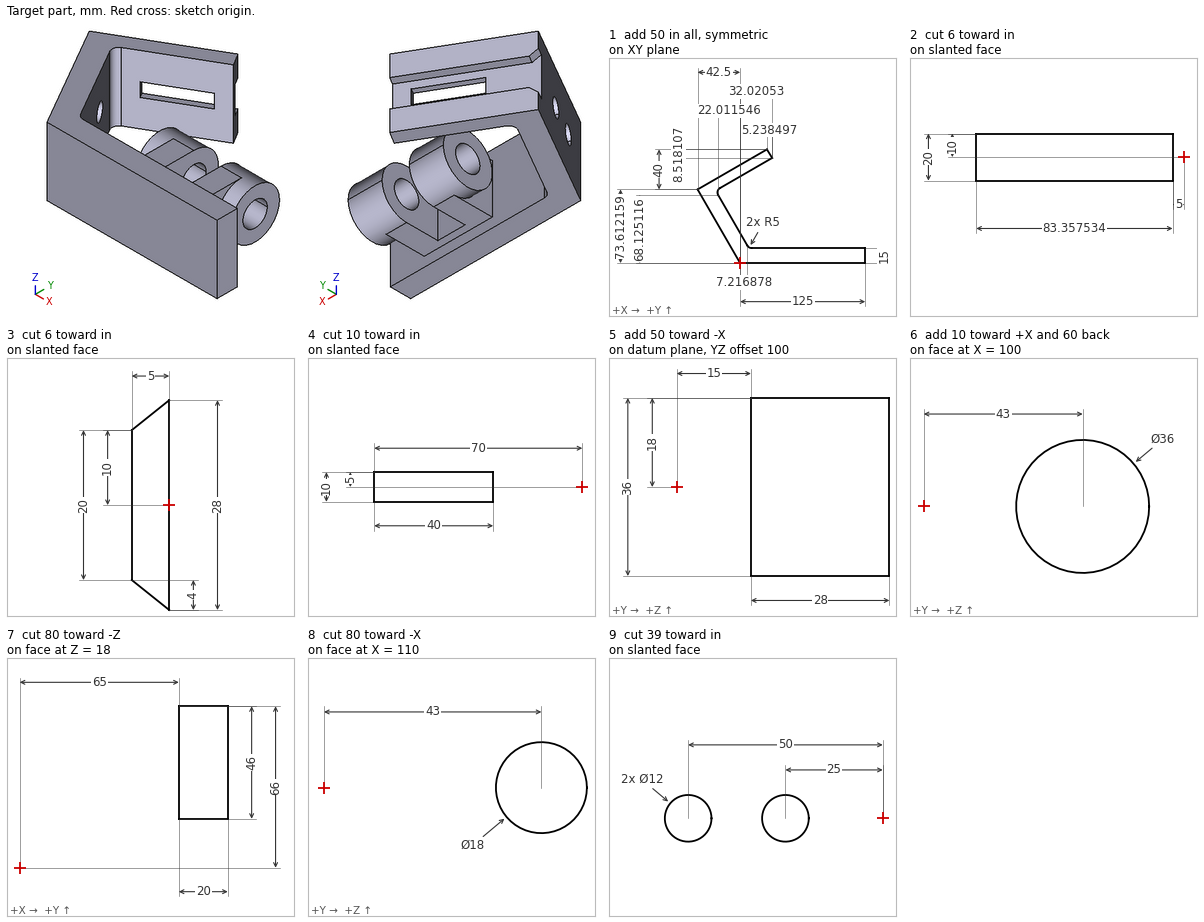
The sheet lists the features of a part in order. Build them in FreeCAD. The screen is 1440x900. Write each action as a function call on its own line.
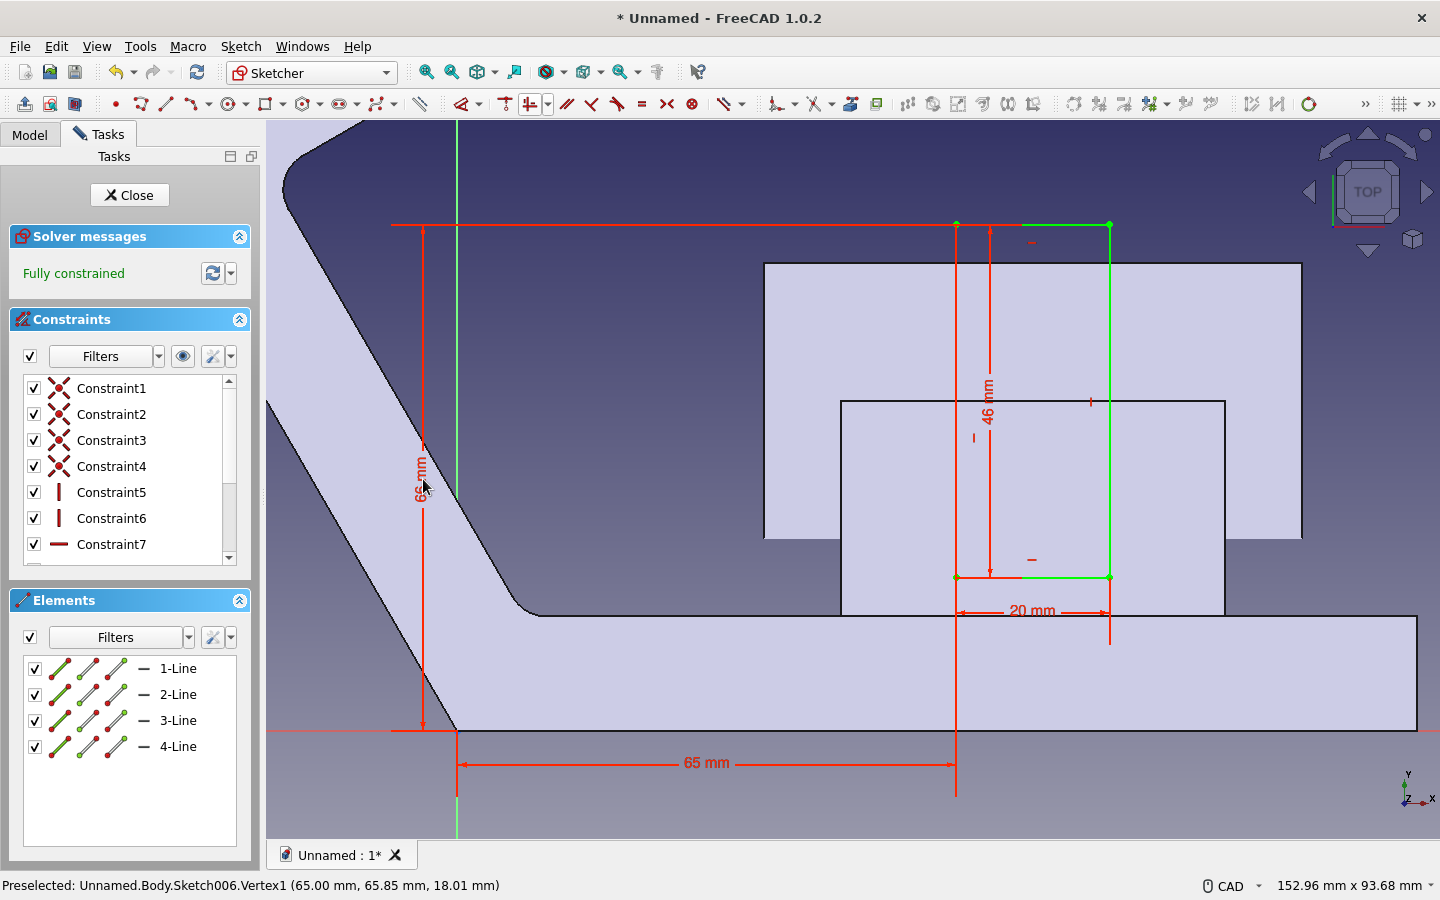
click(130, 195)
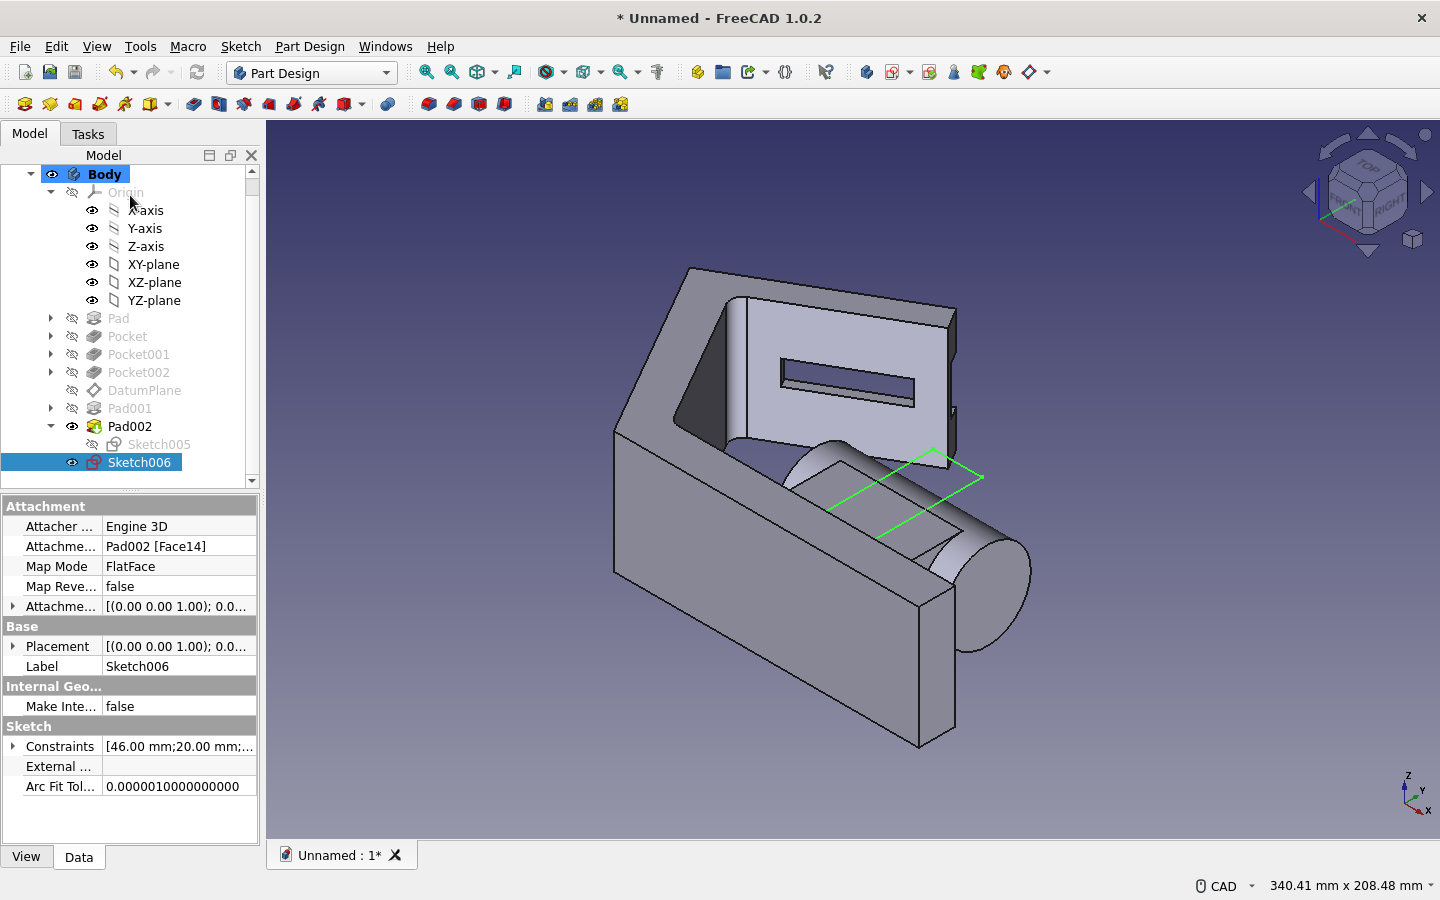
click(194, 104)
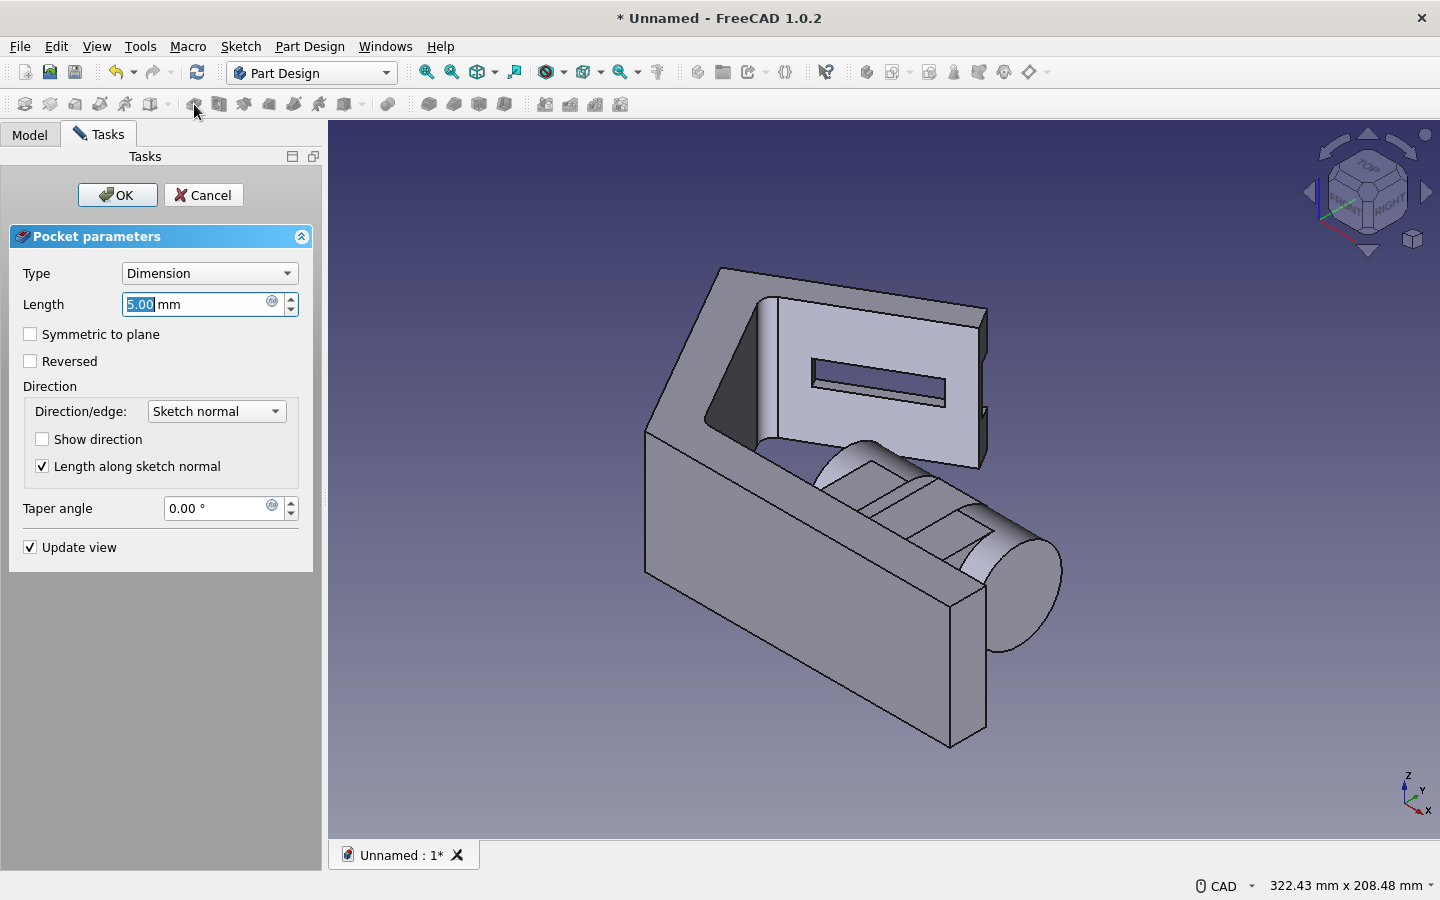
text(80)
key(Tab)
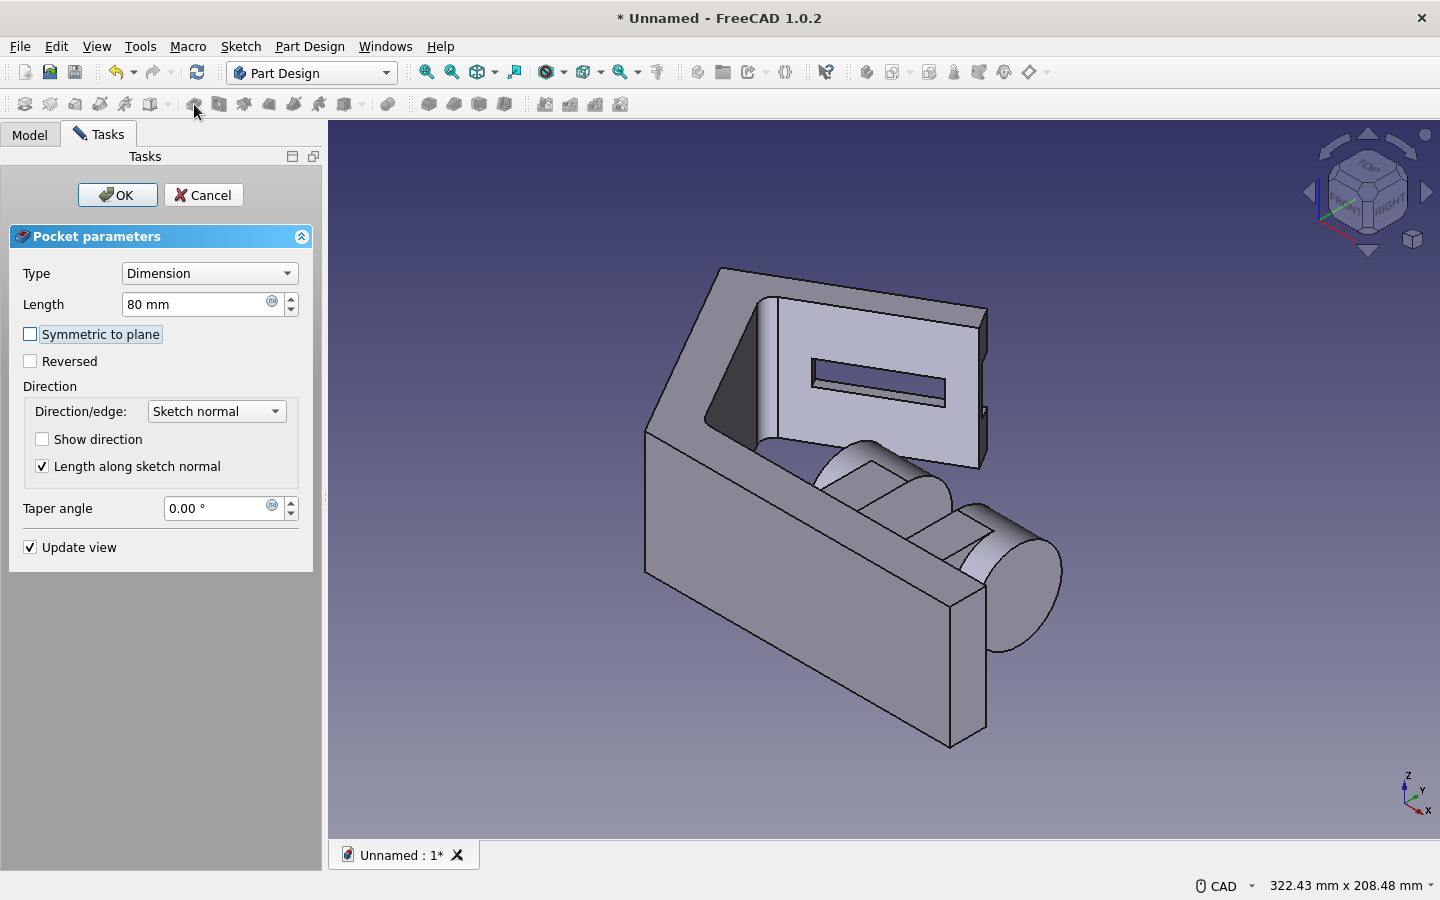
click(118, 195)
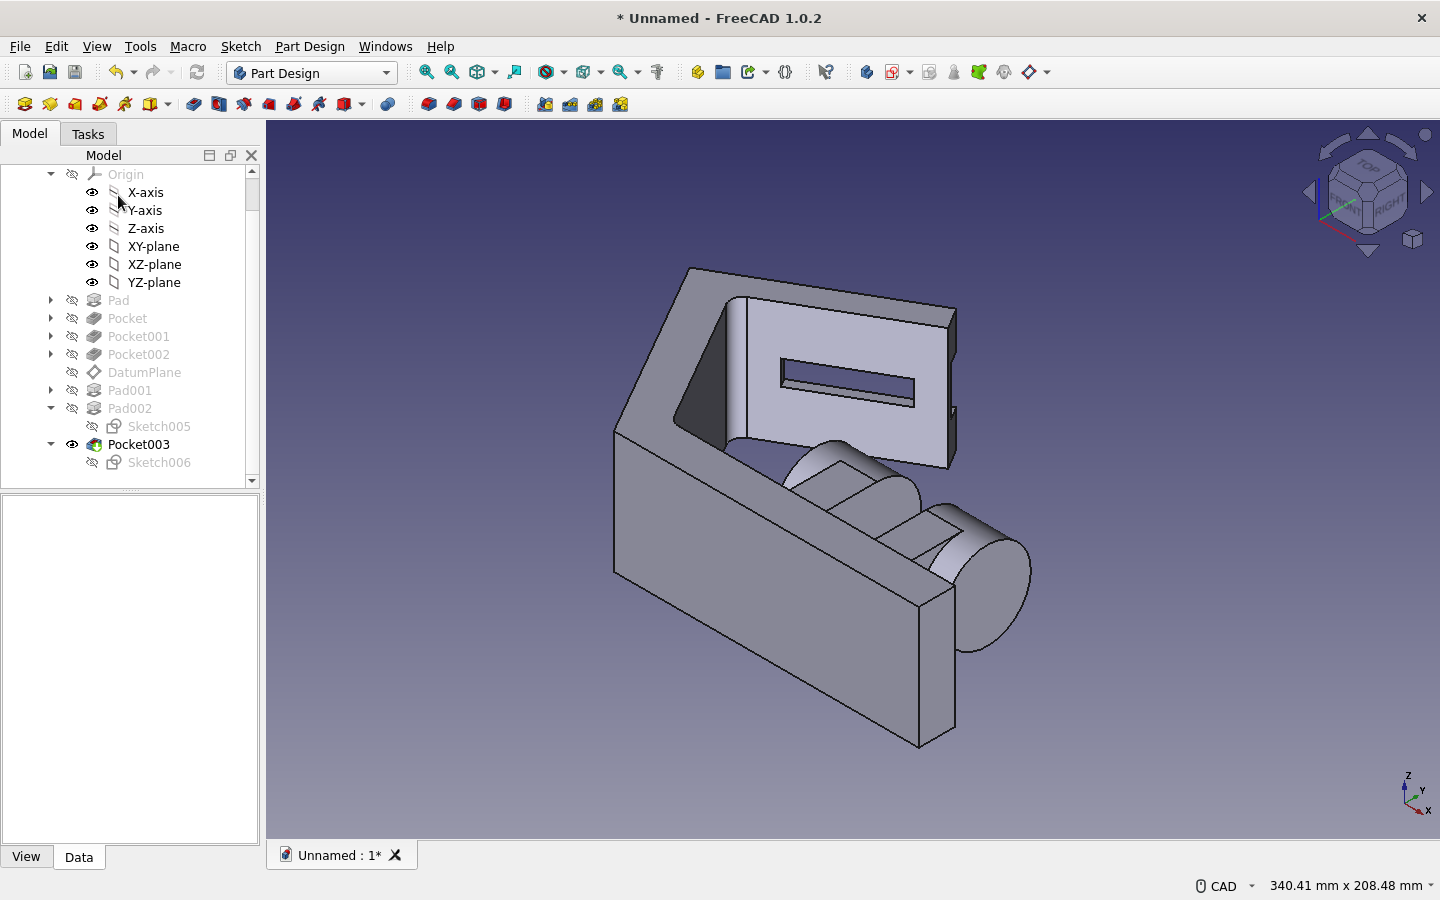
click(987, 595)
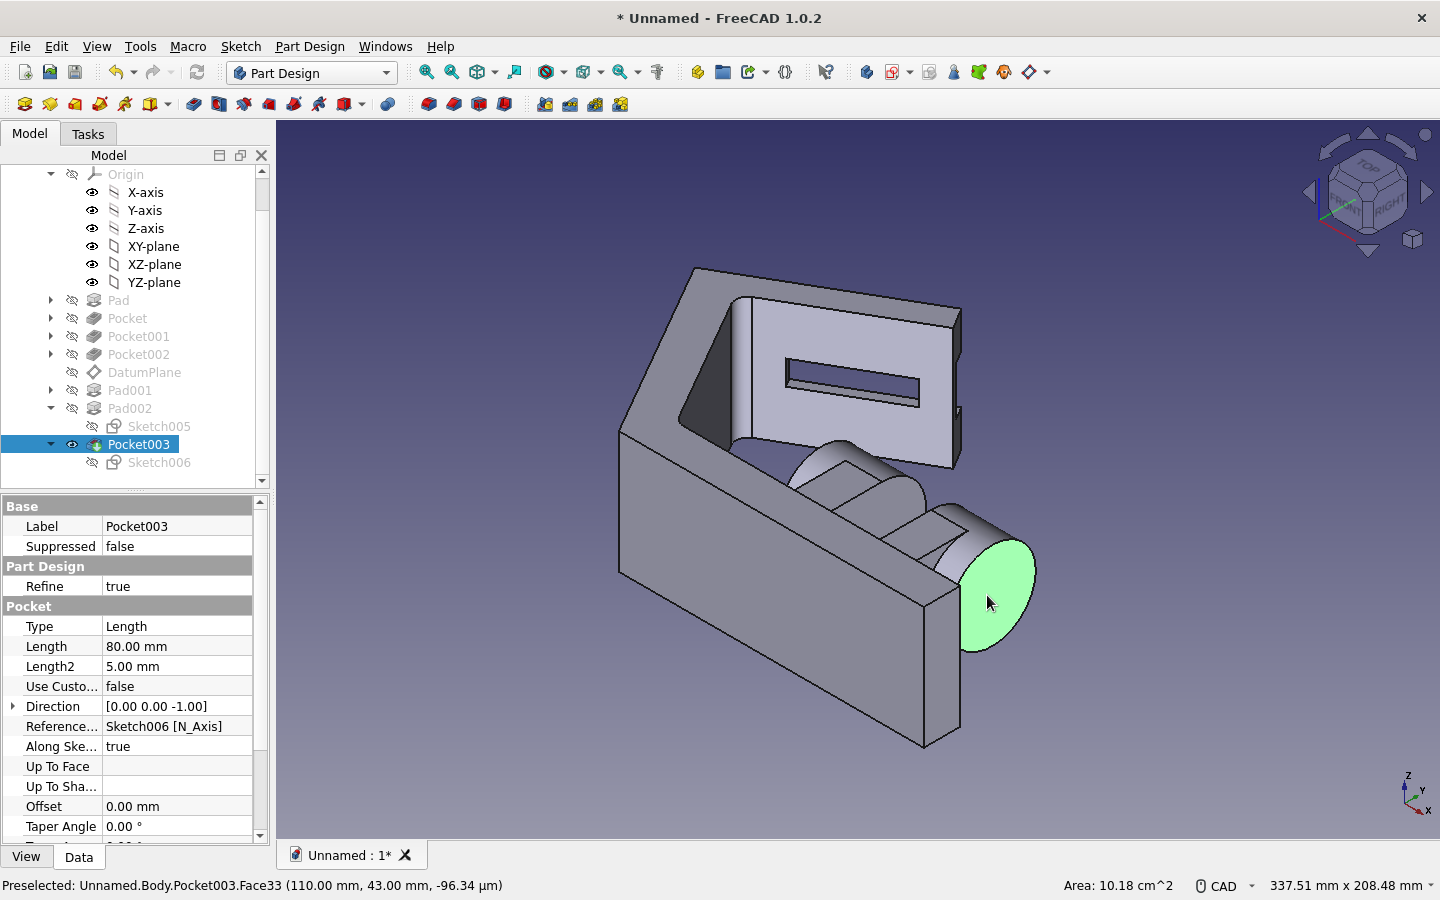
click(892, 72)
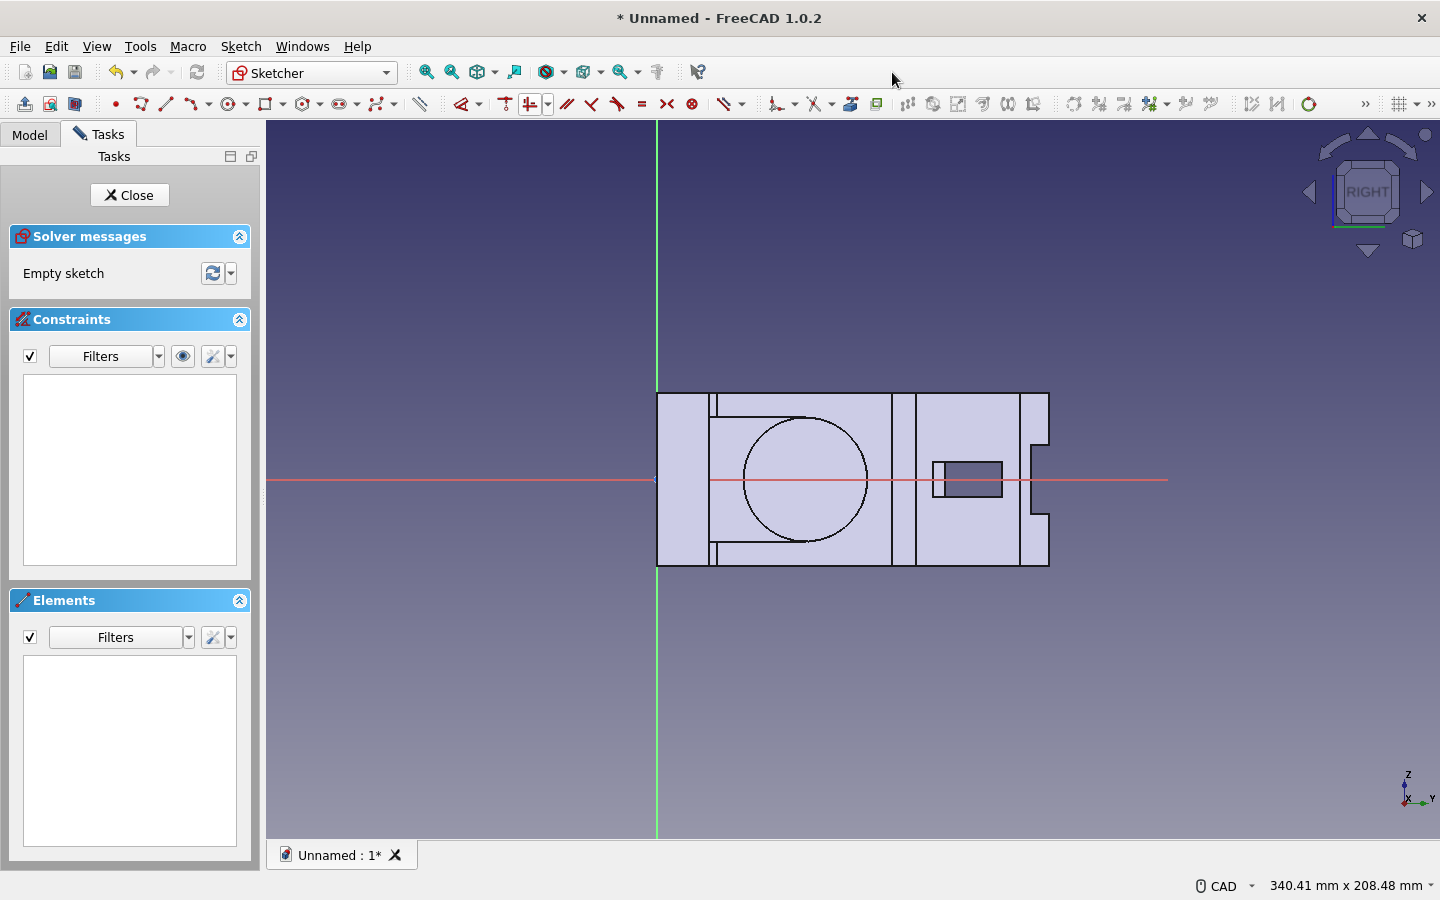
key(q)
key(s)